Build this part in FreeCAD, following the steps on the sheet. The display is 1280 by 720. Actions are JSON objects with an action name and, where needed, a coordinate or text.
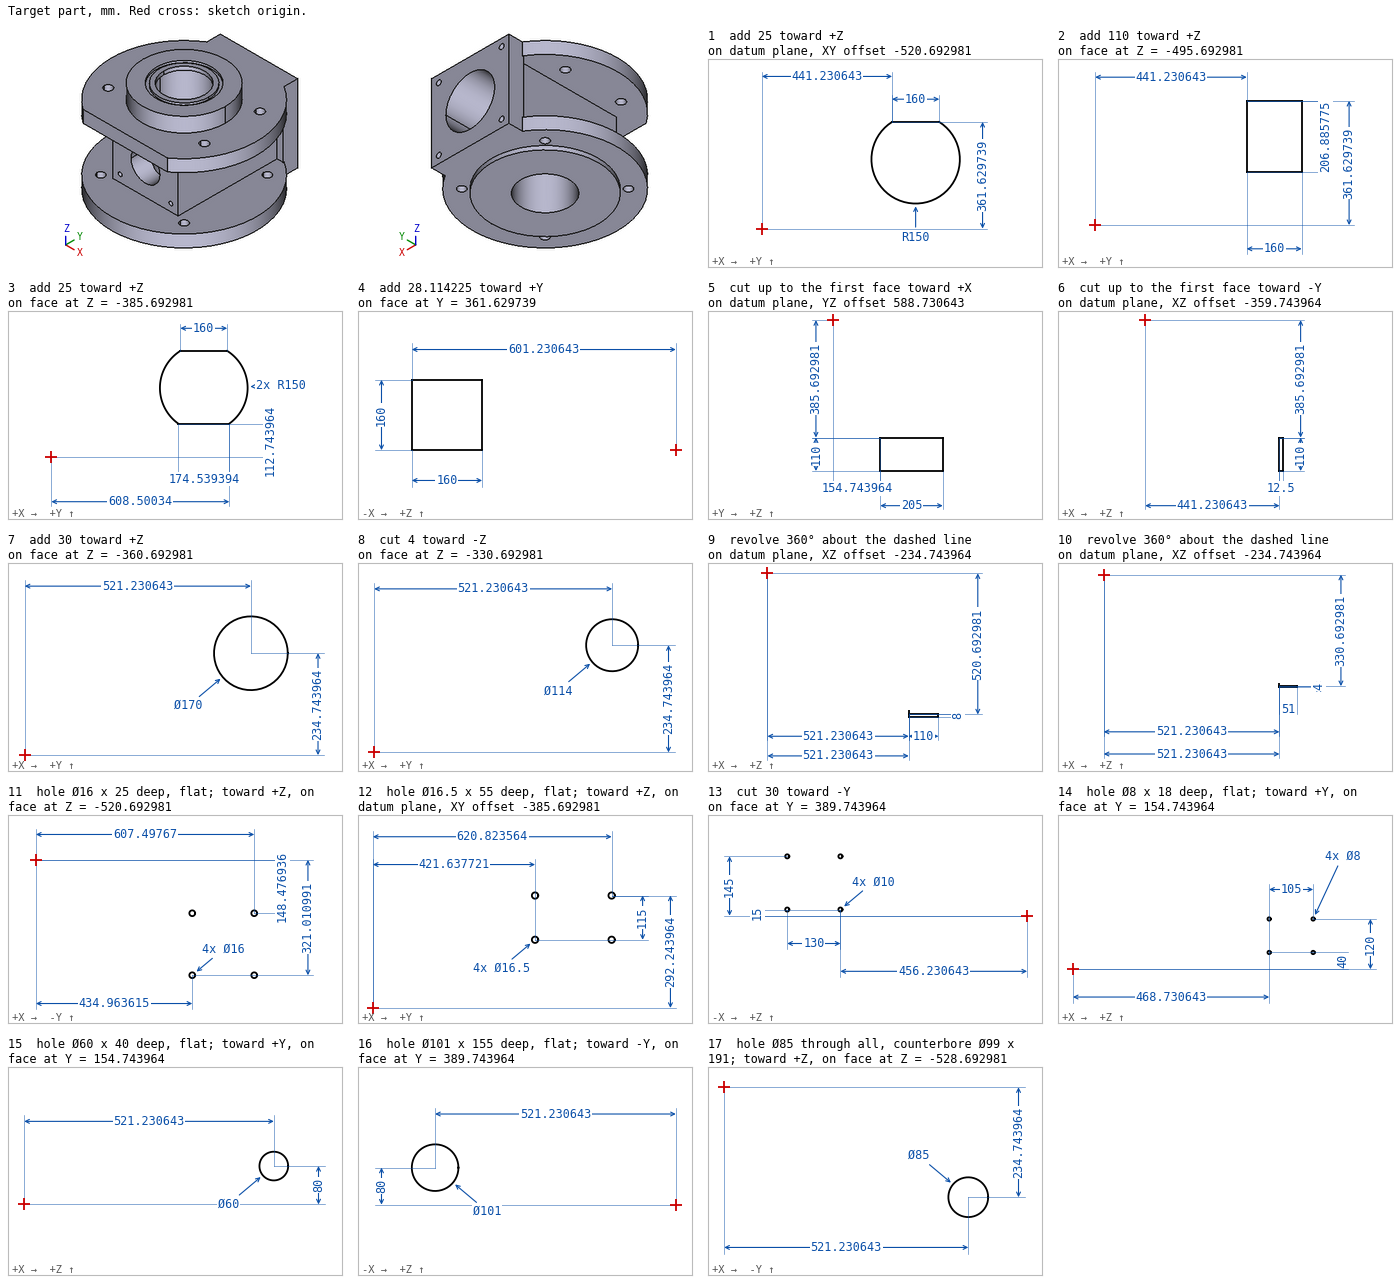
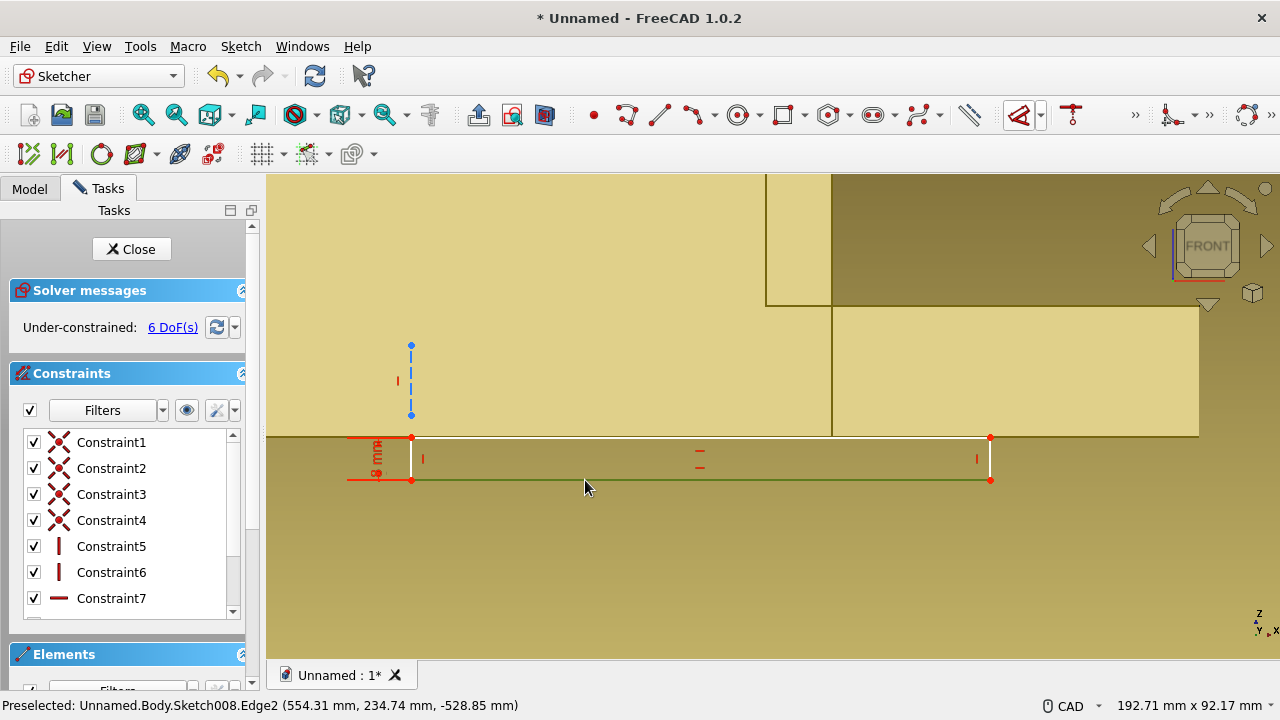
{"action": "left_click", "coordinate": [1040, 116]}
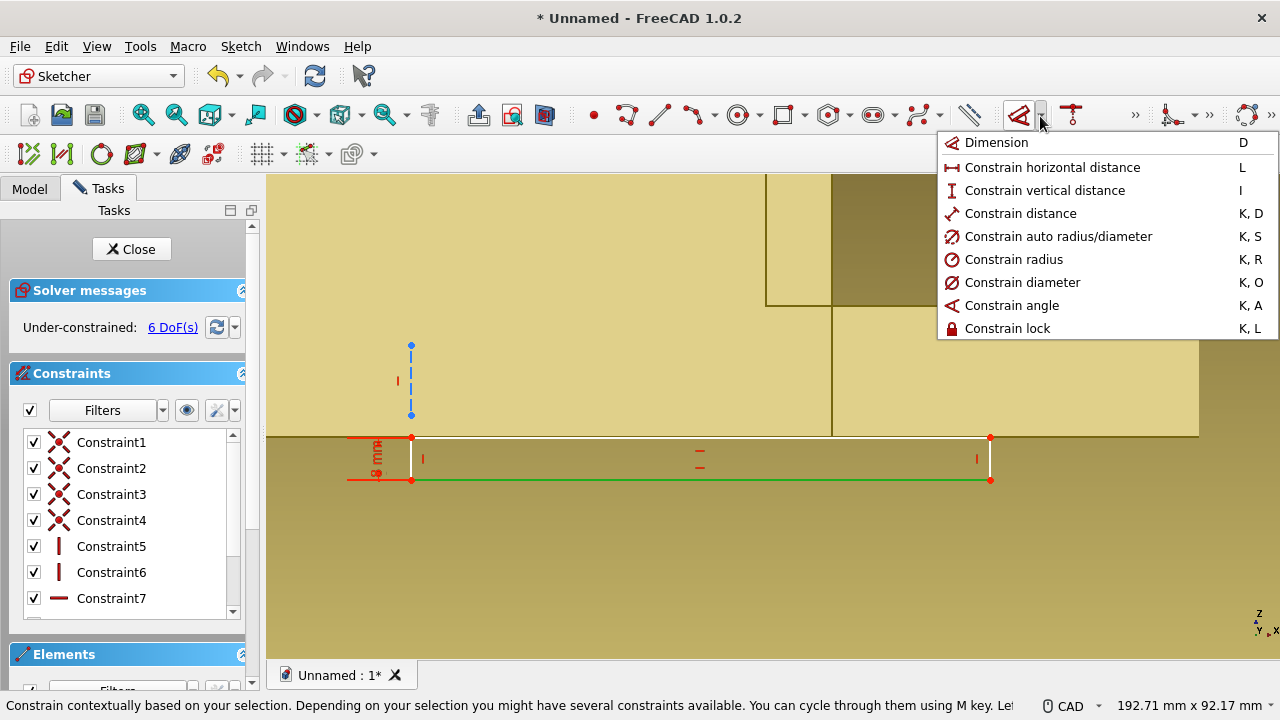
{"action": "left_click", "coordinate": [1108, 168]}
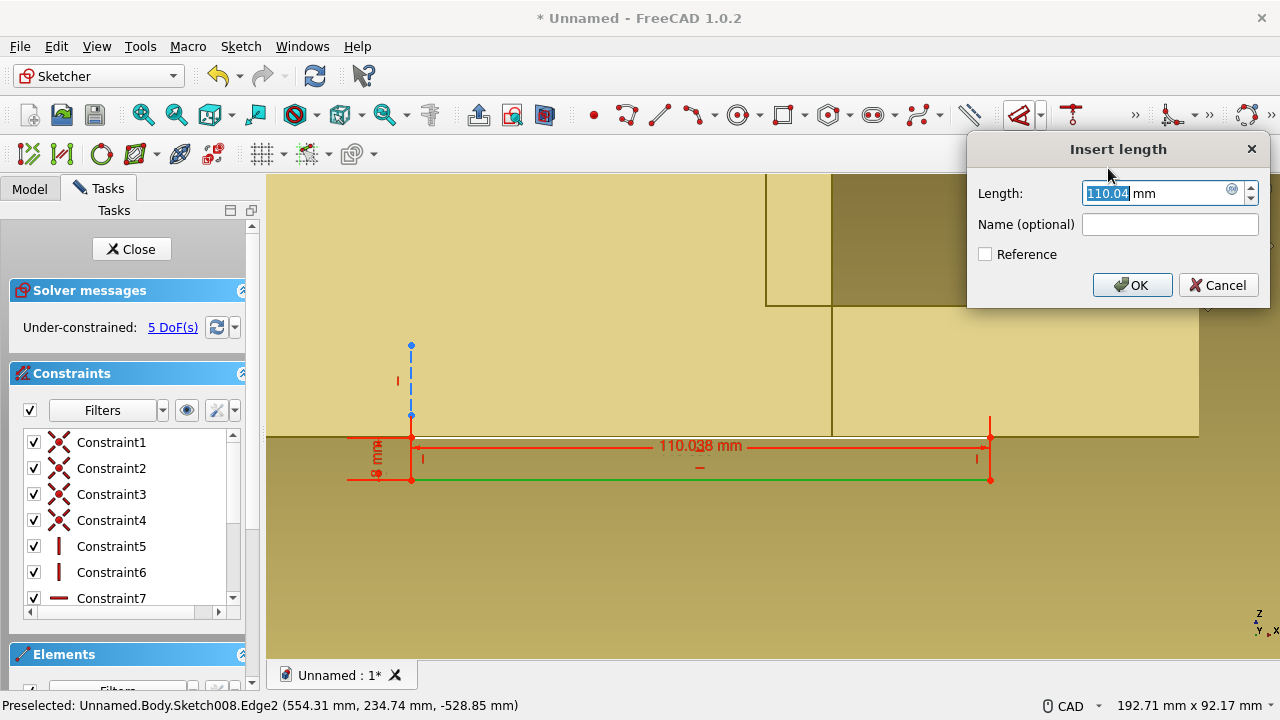
{"action": "type", "text": "110"}
{"action": "key", "text": "Return"}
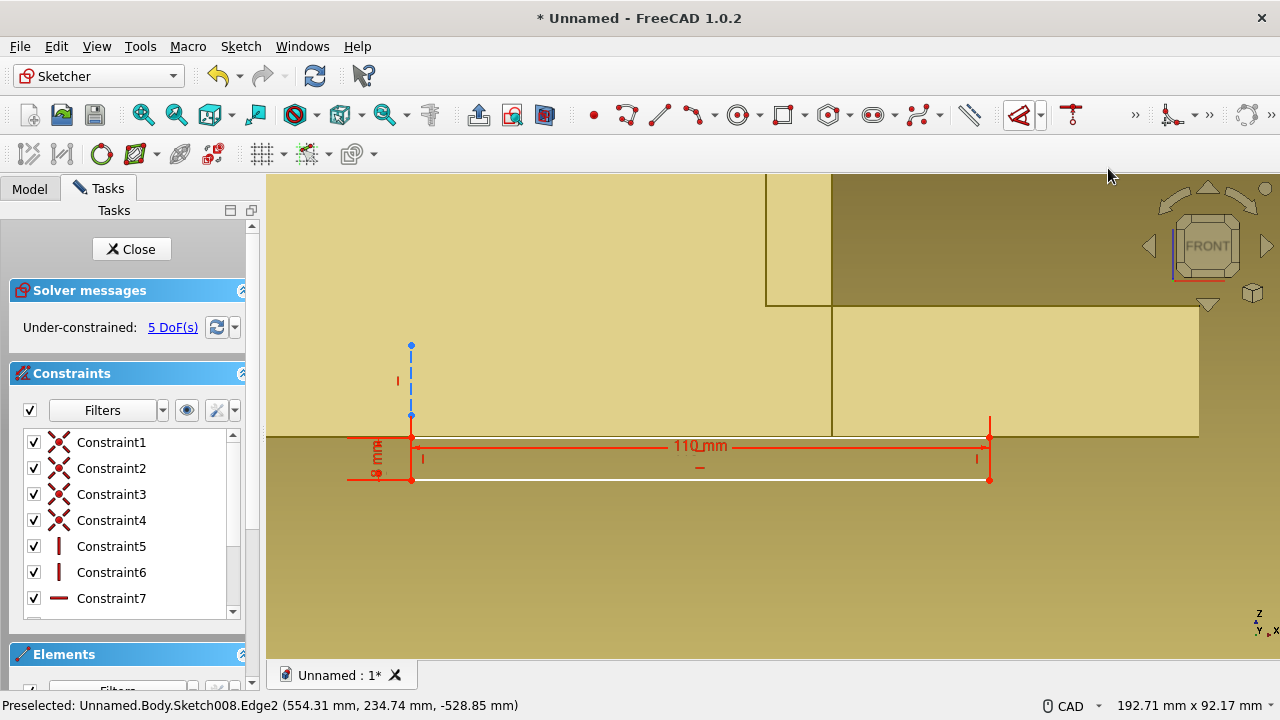
{"action": "left_click", "coordinate": [411, 438]}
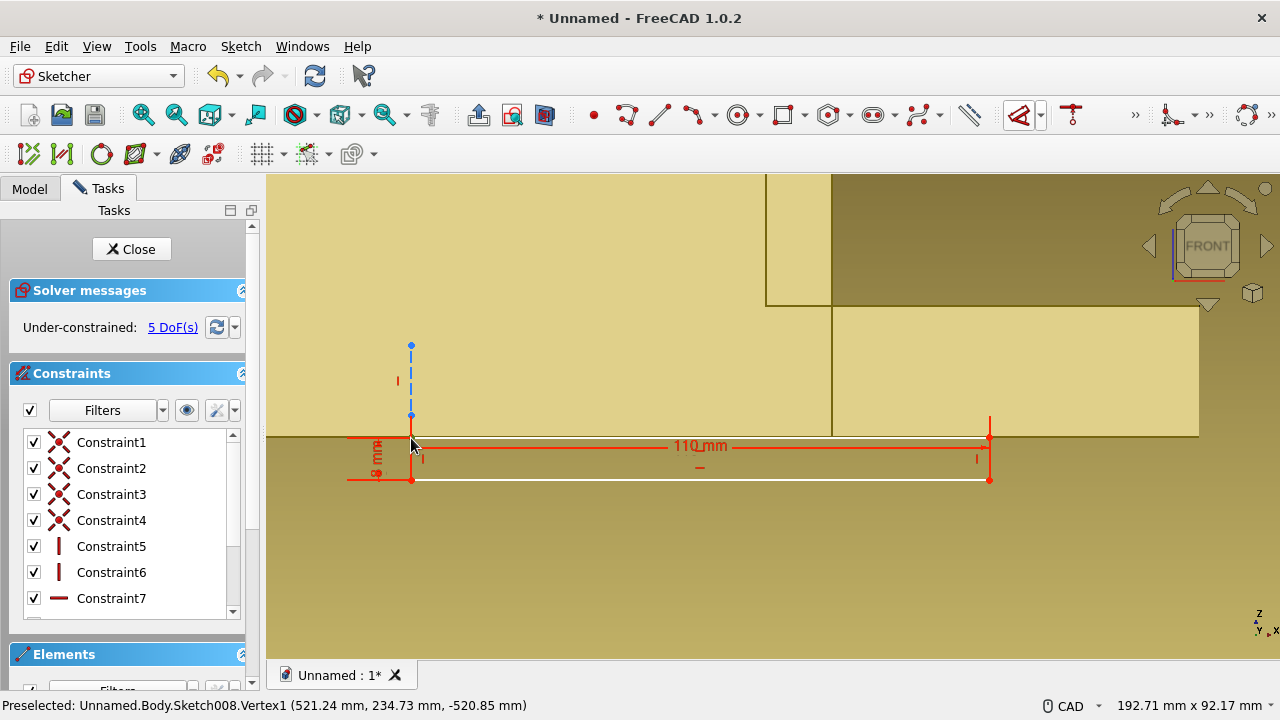
{"action": "key", "text": "l"}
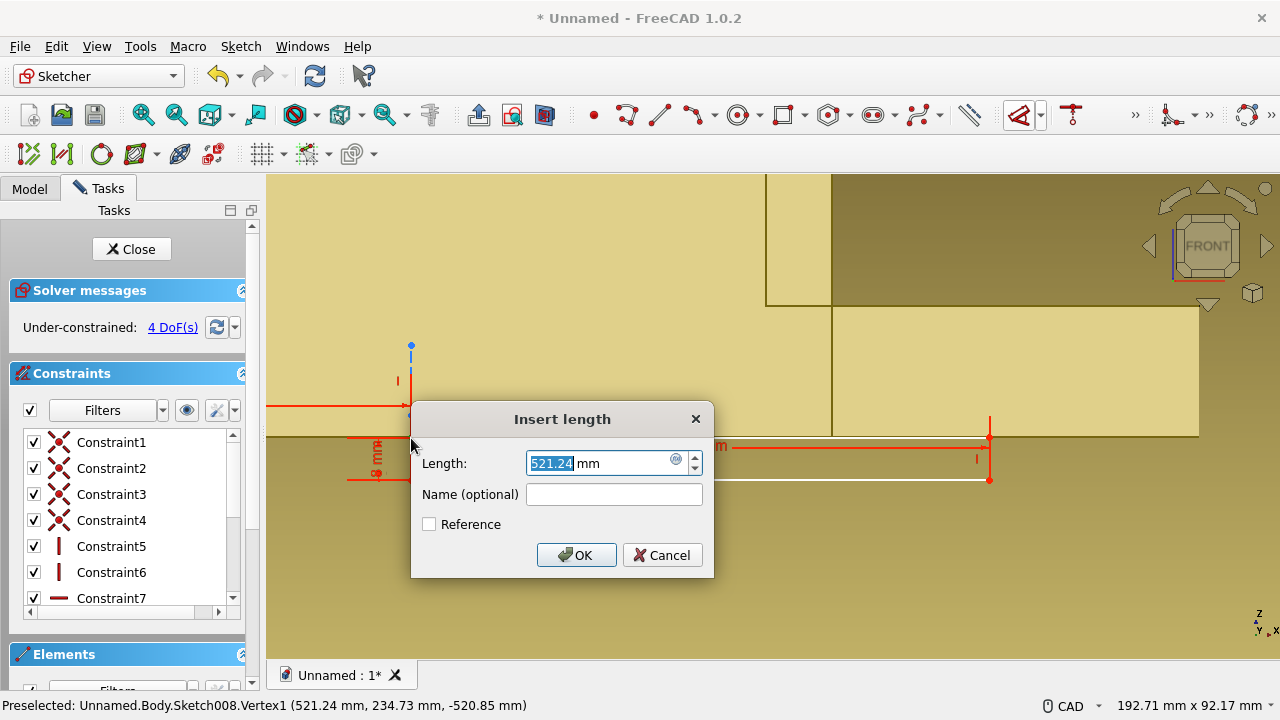
{"action": "type", "text": "521.230643"}
{"action": "key", "text": "Return"}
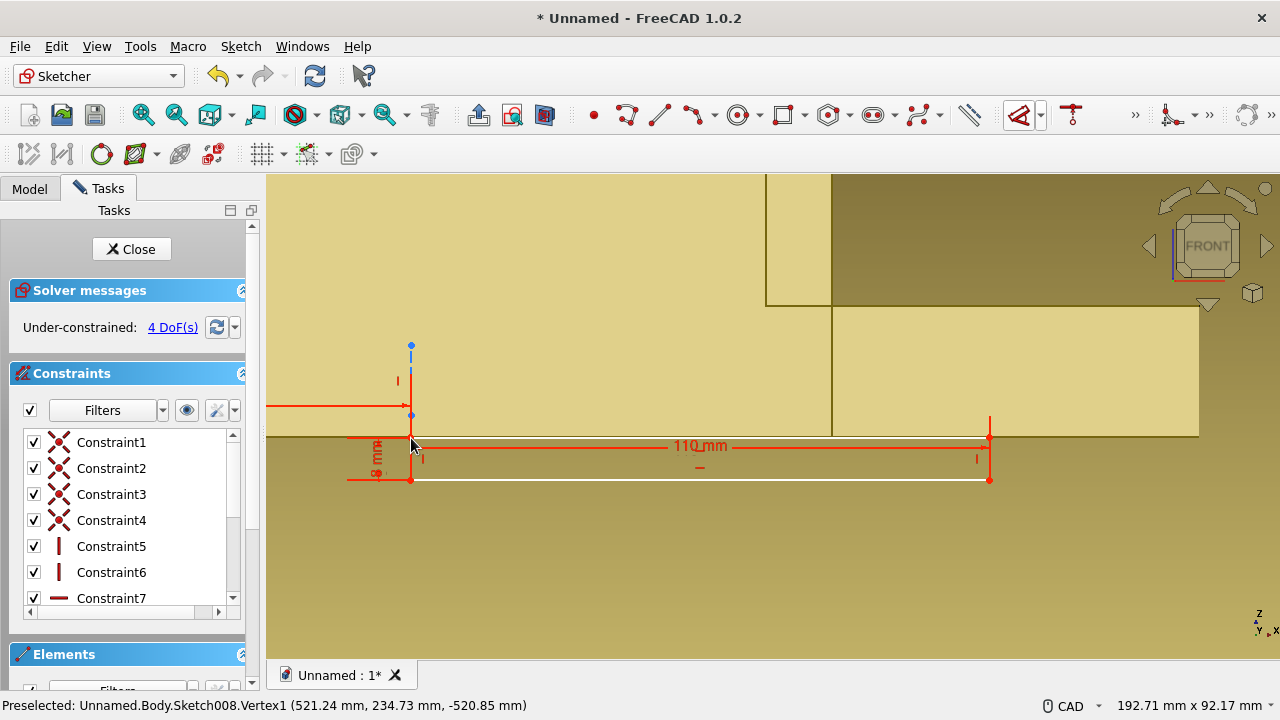
{"action": "left_click", "coordinate": [411, 438]}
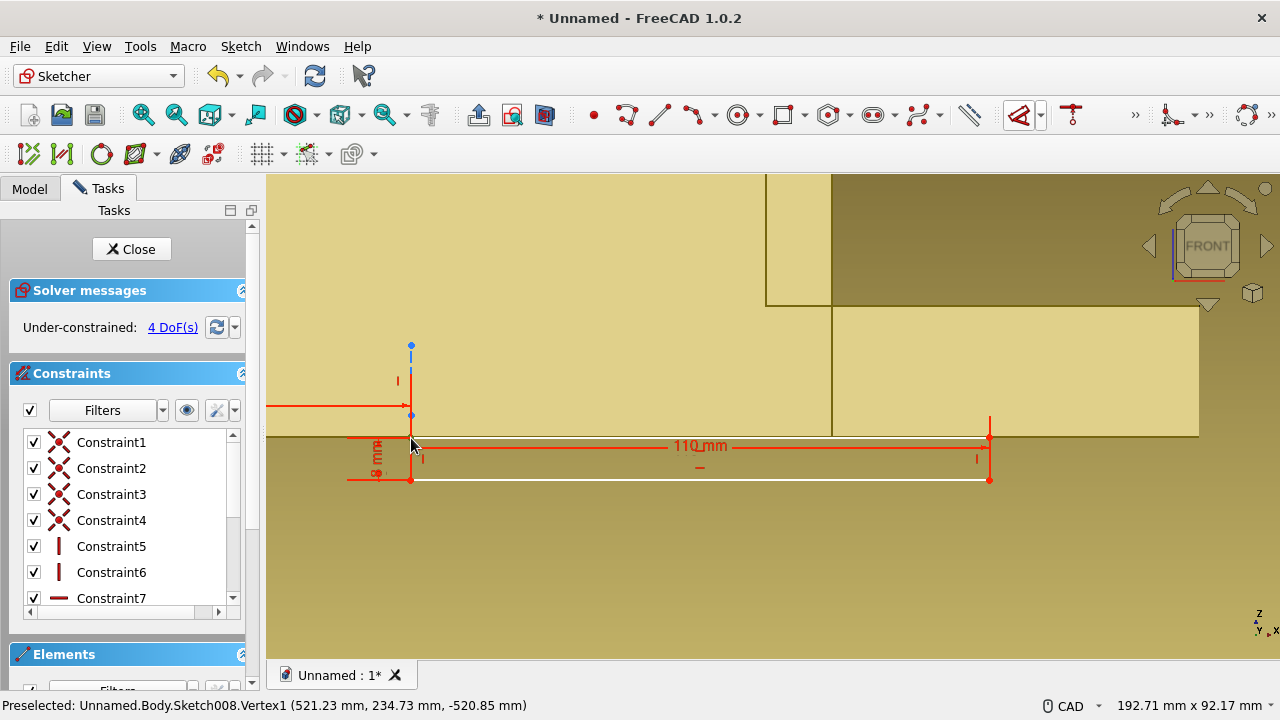
{"action": "left_click", "coordinate": [1040, 116]}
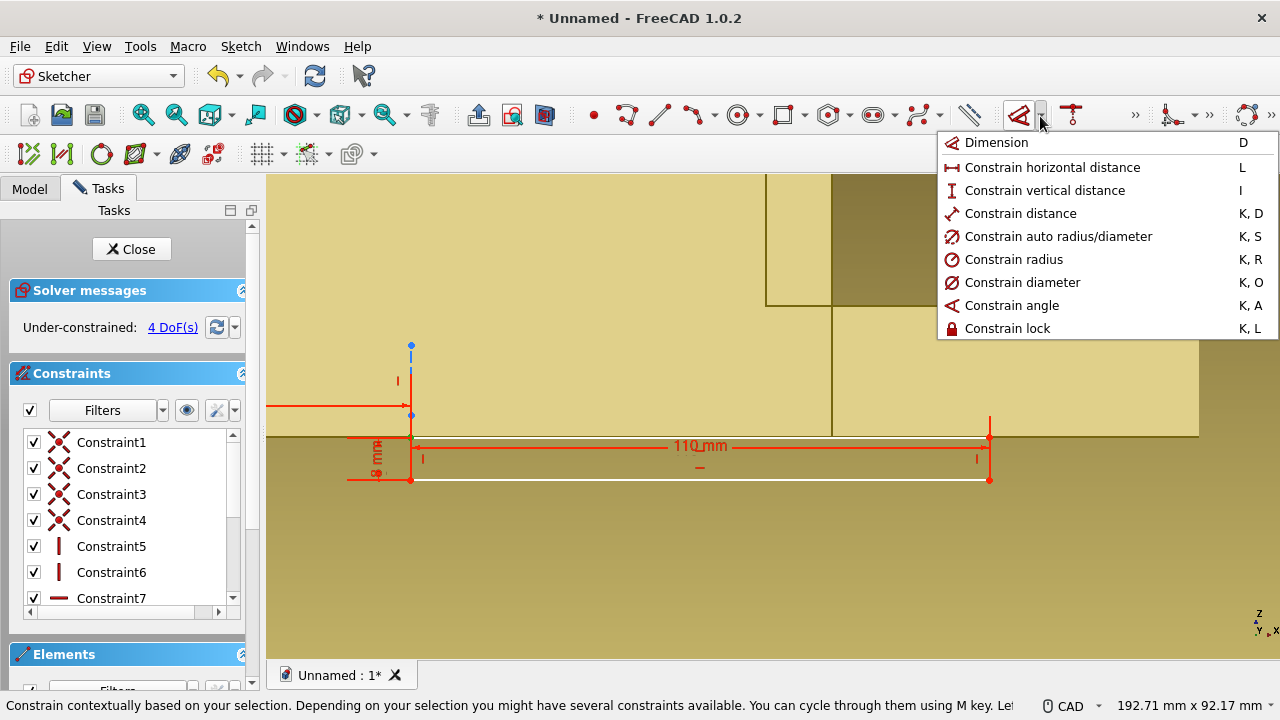
{"action": "left_click", "coordinate": [1108, 190]}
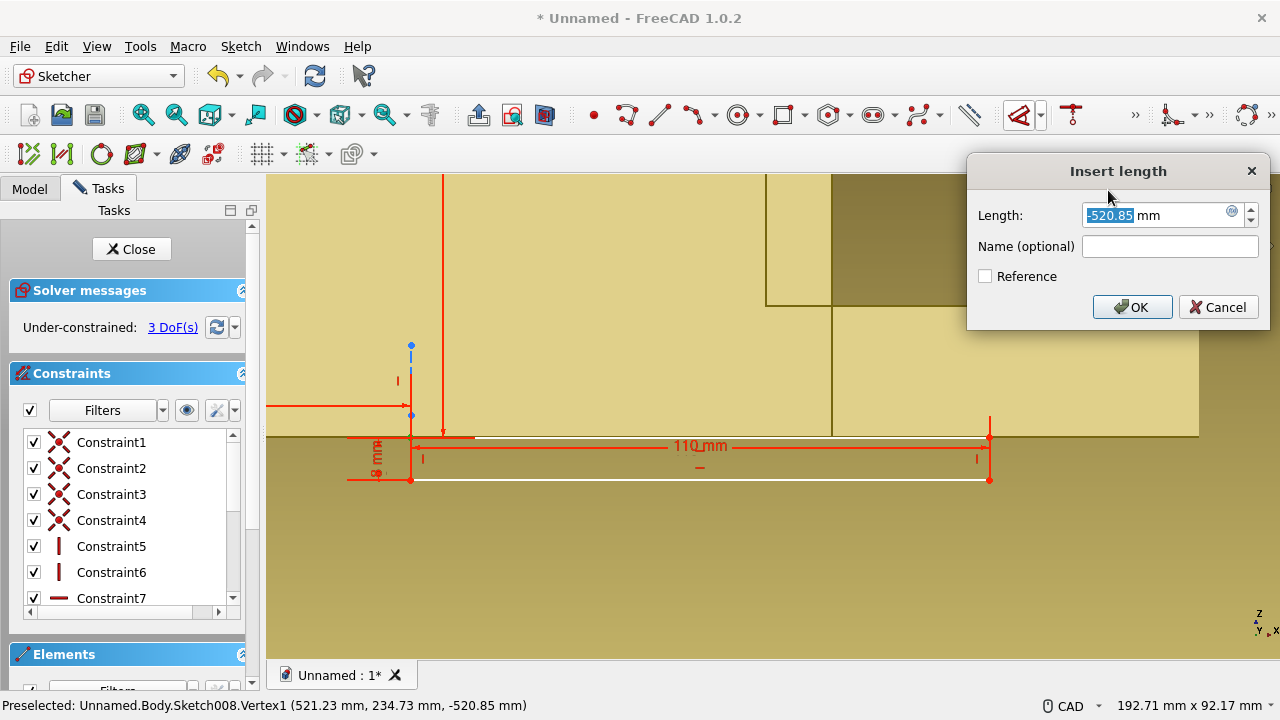
{"action": "type", "text": "-520.692981"}
{"action": "key", "text": "Return"}